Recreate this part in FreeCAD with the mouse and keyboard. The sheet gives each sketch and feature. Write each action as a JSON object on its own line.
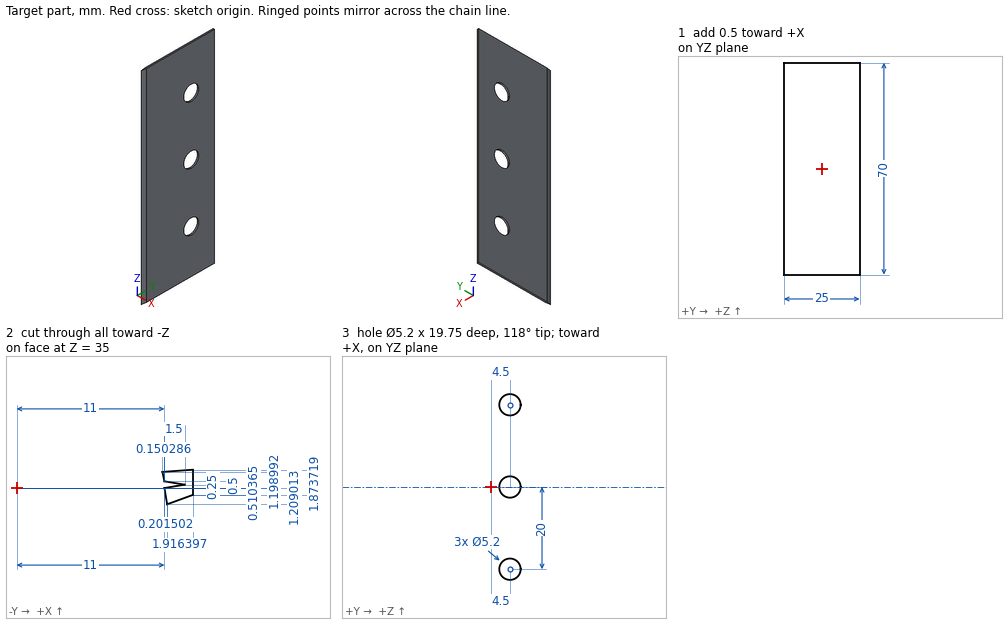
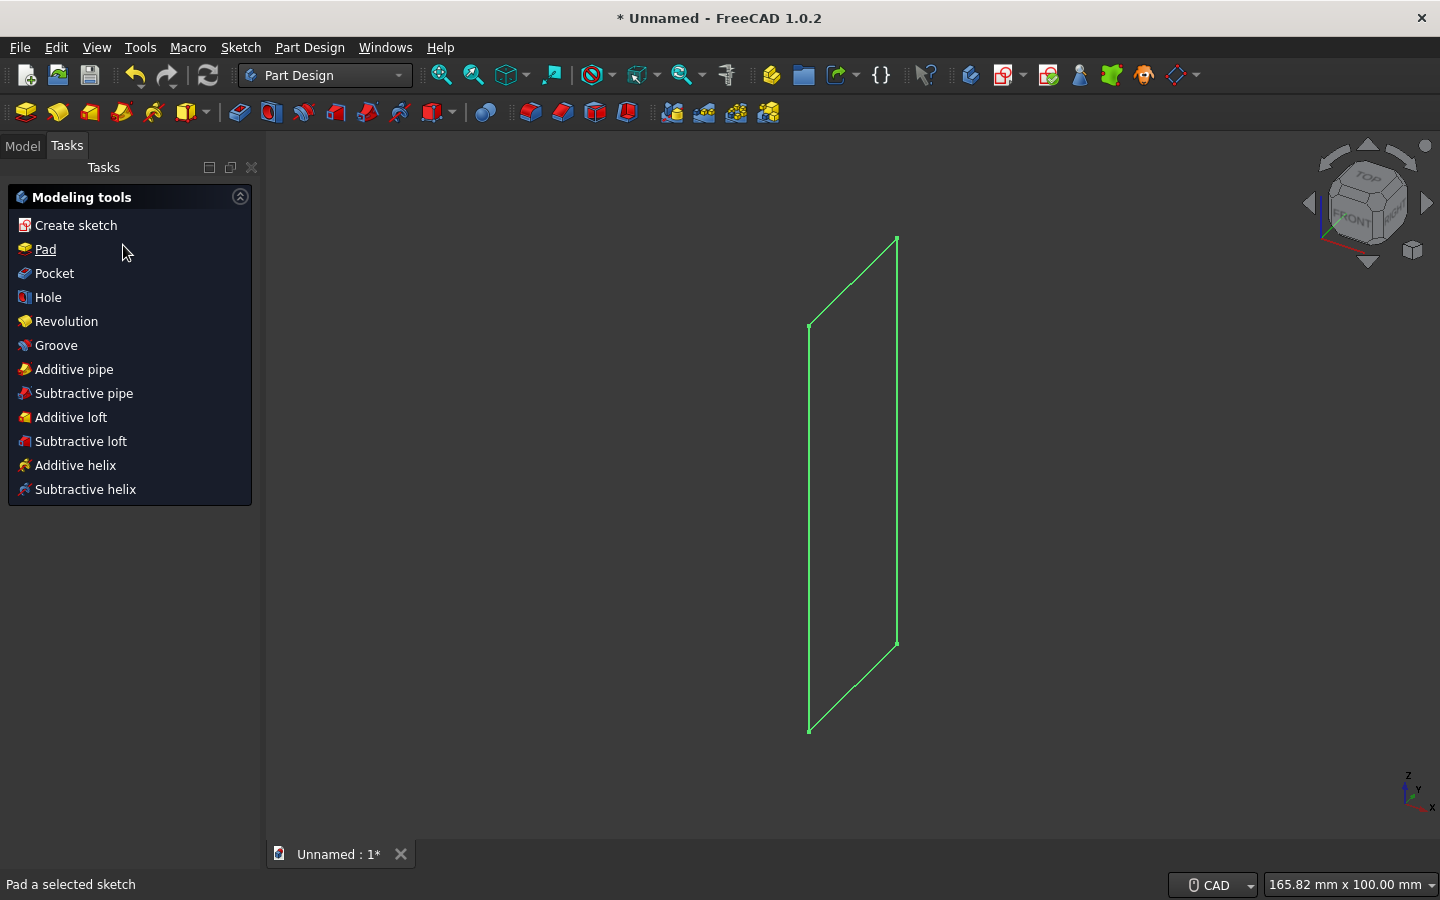
{"action": "left_click", "coordinate": [26, 112]}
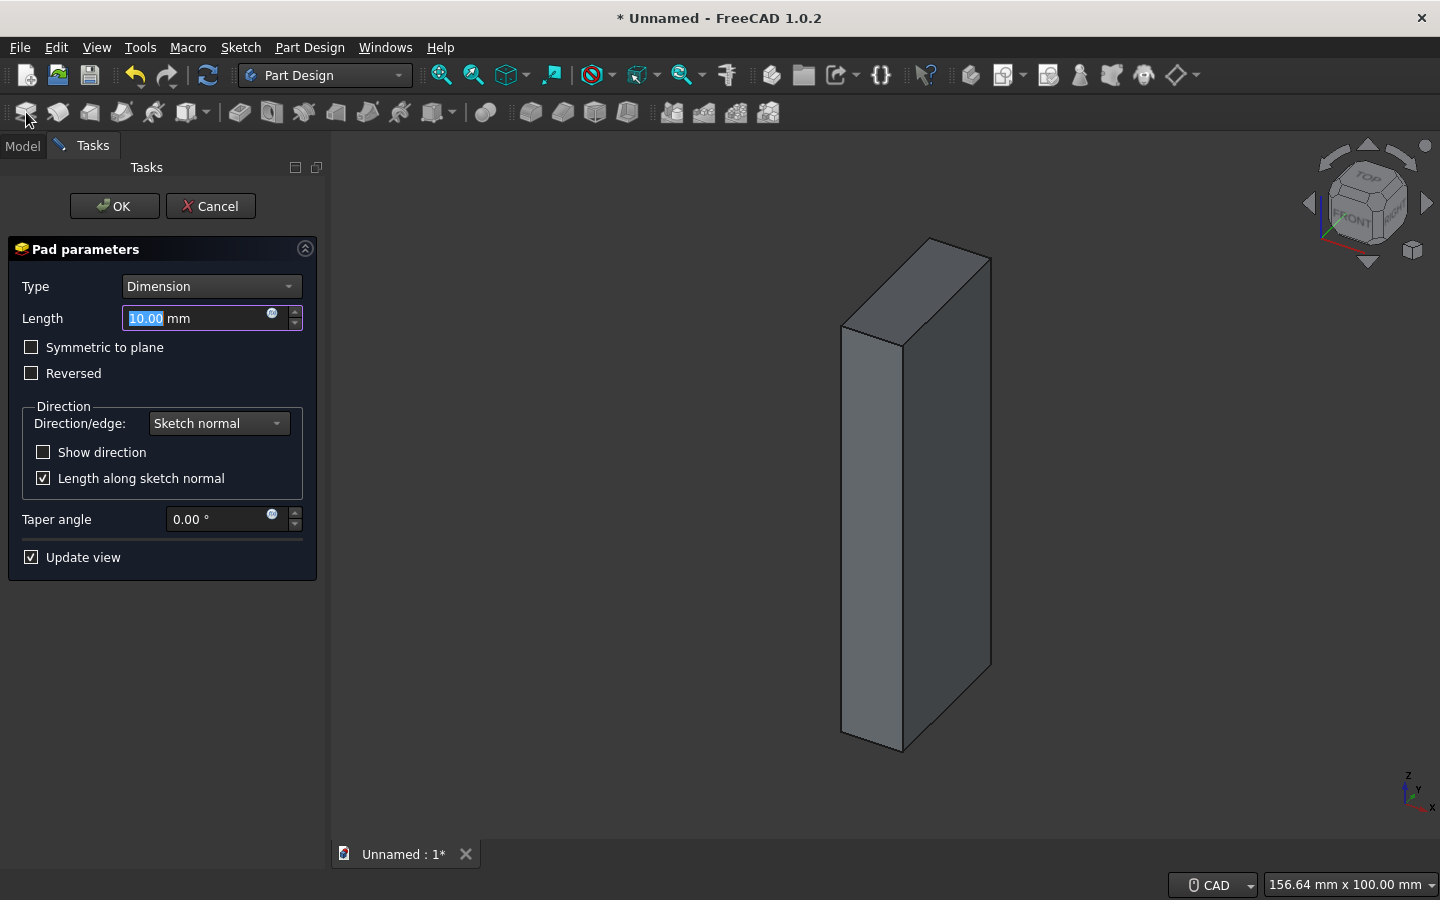
{"action": "type", "text": "0.5"}
{"action": "key", "text": "Tab"}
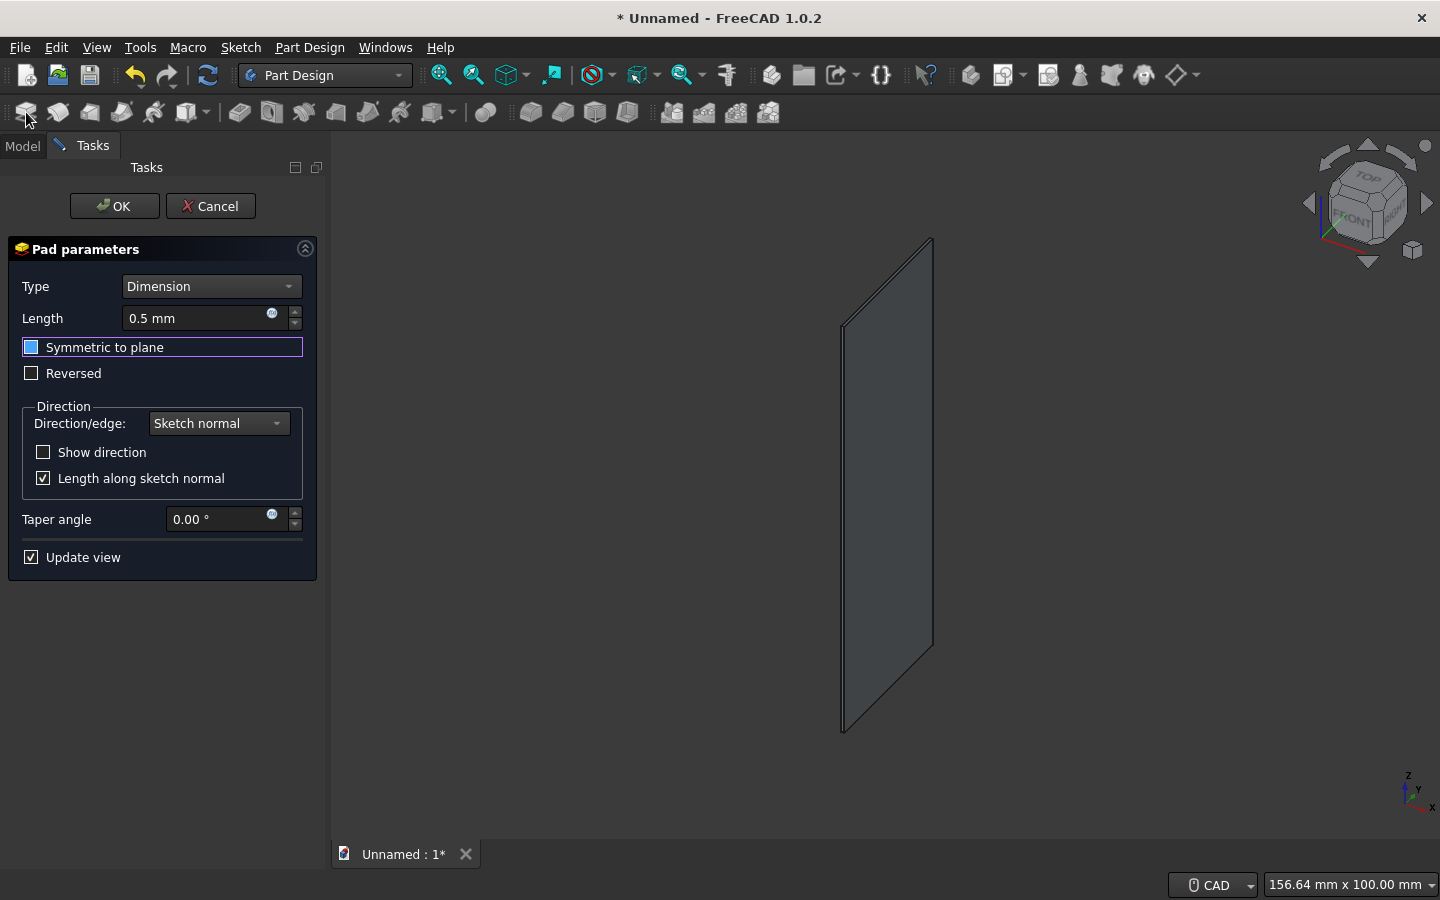
{"action": "left_click", "coordinate": [115, 206]}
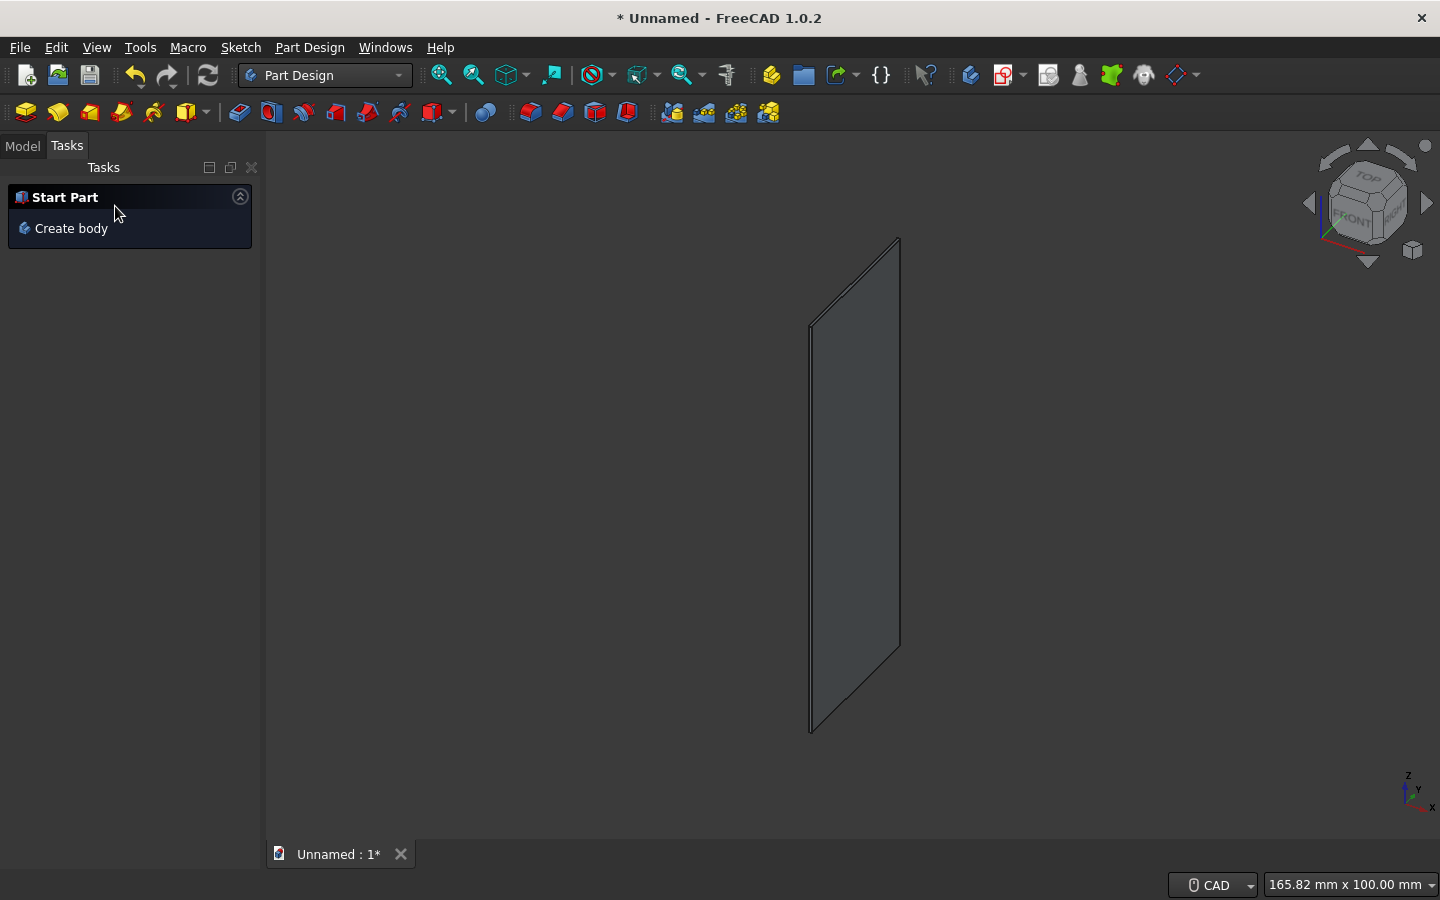
{"action": "scroll", "coordinate": [892, 244], "scroll_direction": "up", "scroll_amount": 10}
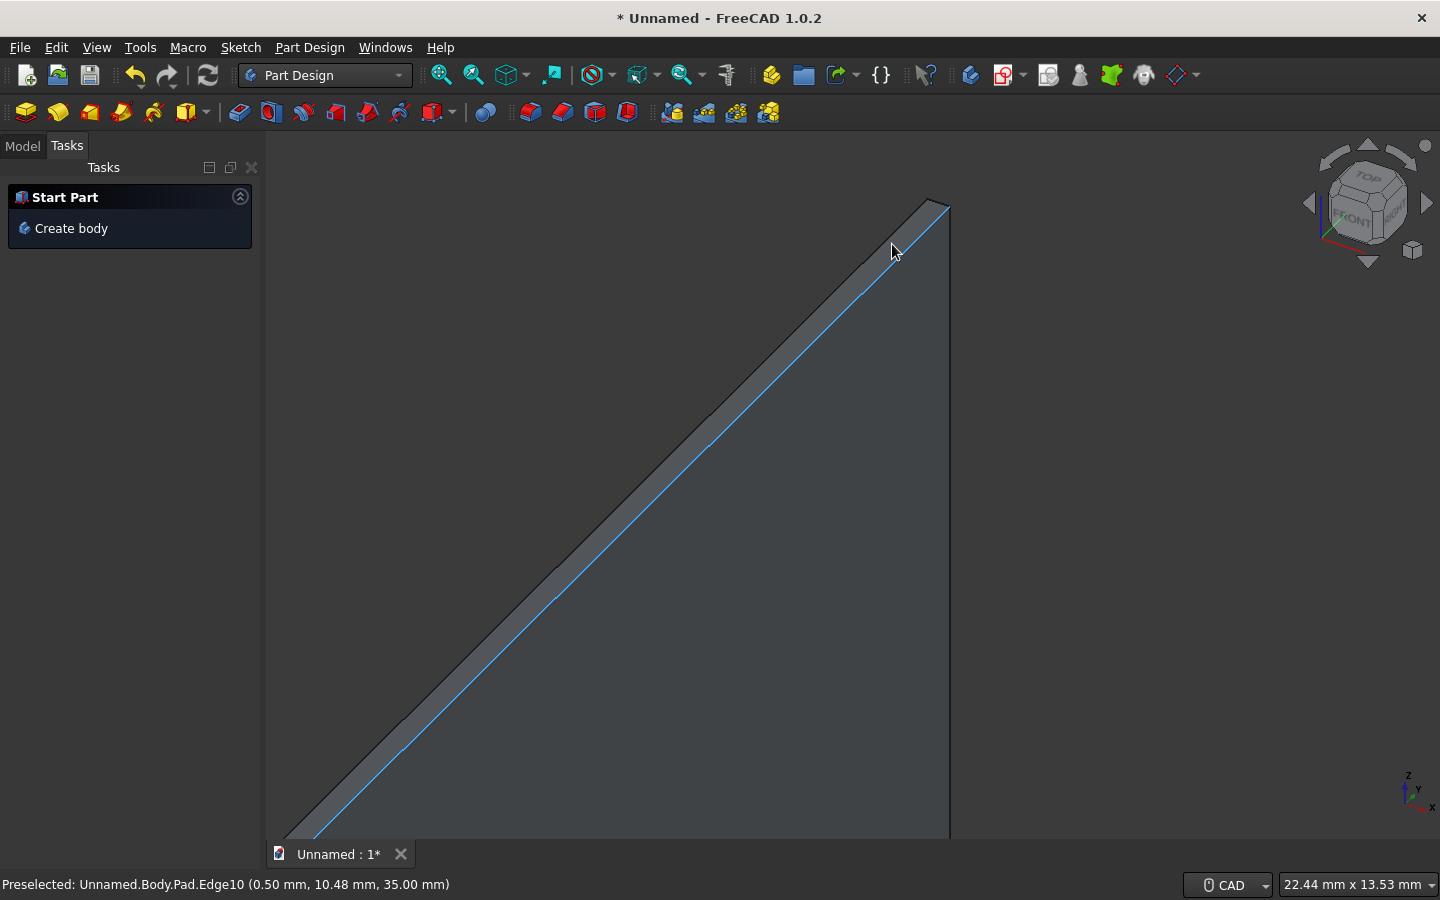
{"action": "left_click", "coordinate": [892, 248]}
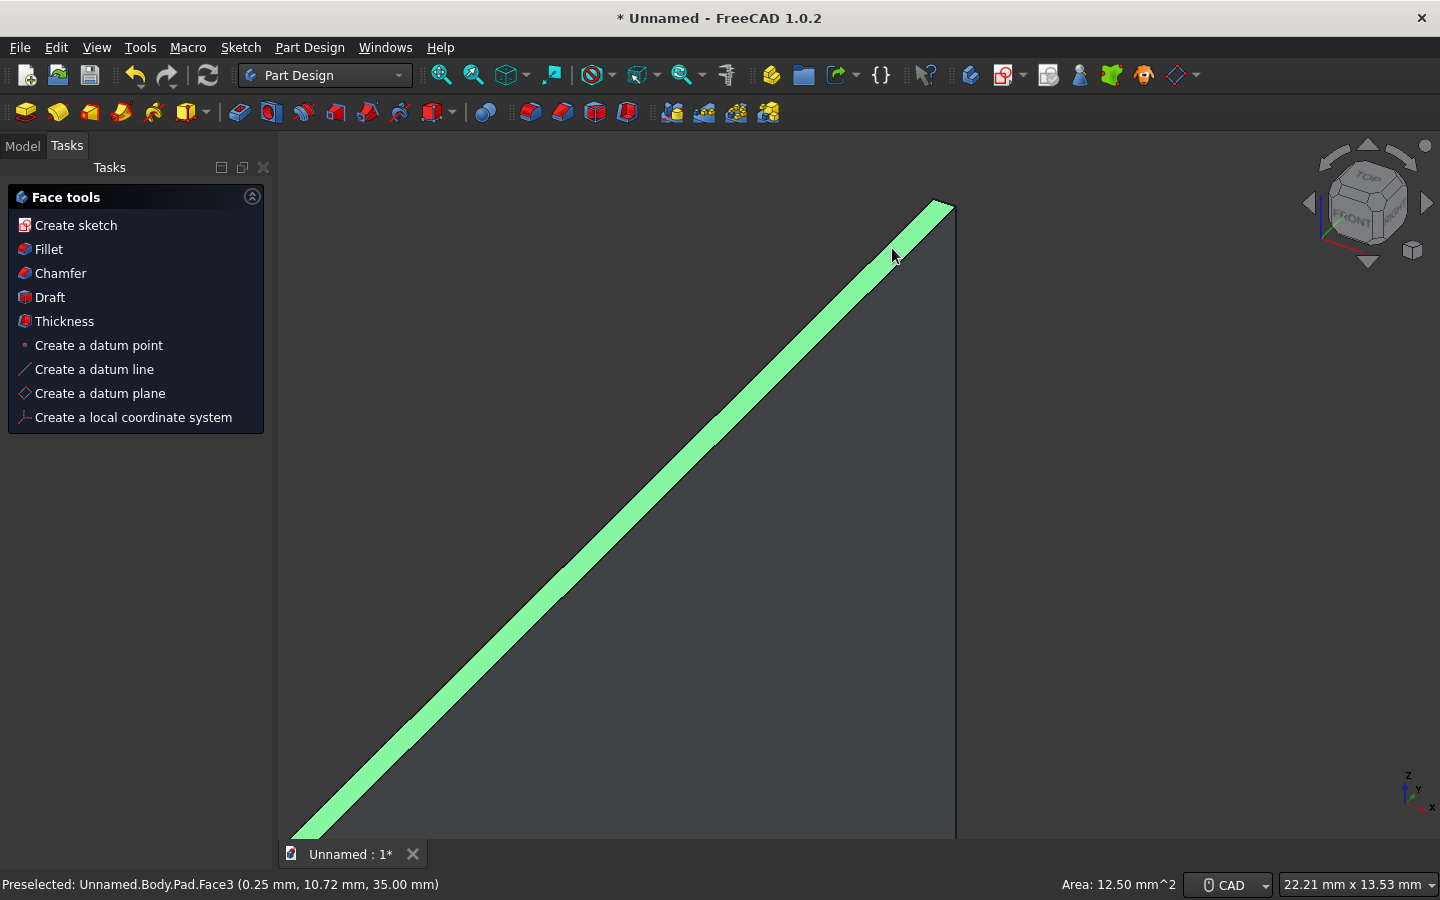
{"action": "left_click", "coordinate": [1004, 76]}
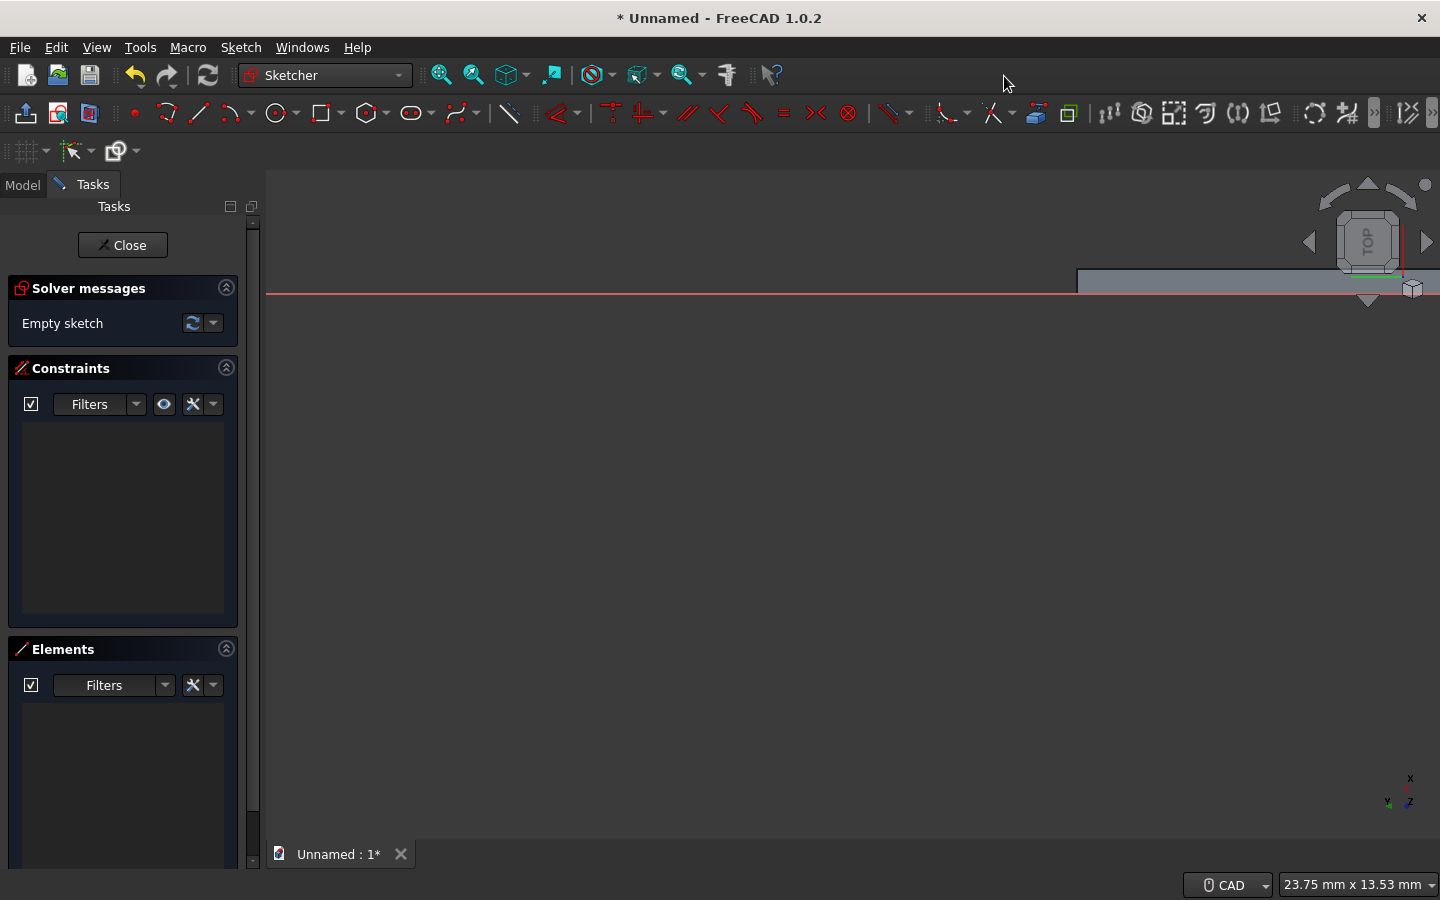
{"action": "scroll", "coordinate": [784, 504], "scroll_direction": "down", "scroll_amount": 5}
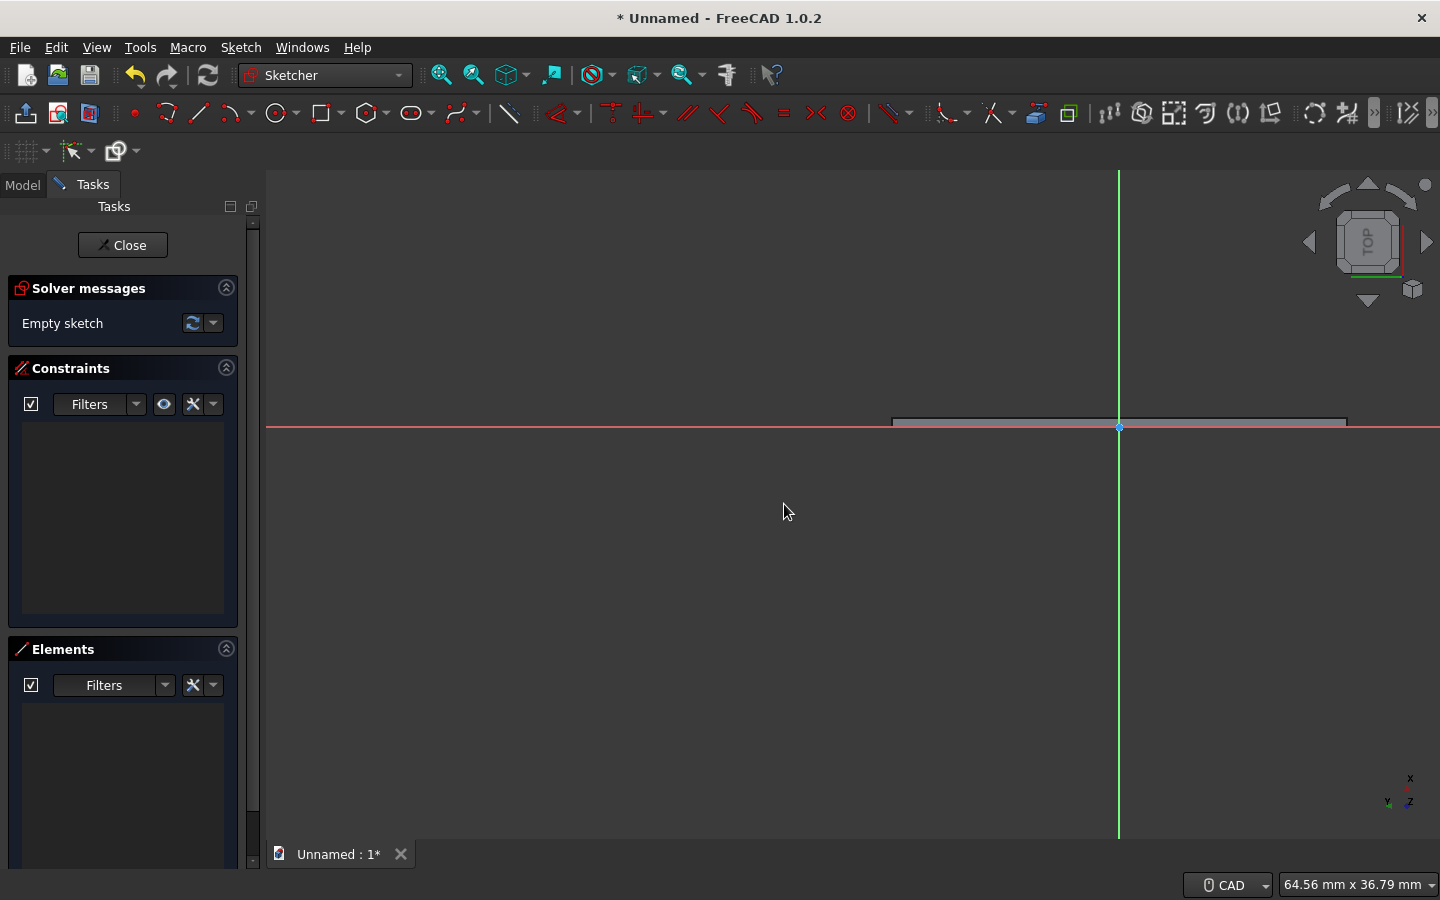
{"action": "scroll", "coordinate": [784, 504], "scroll_direction": "down", "scroll_amount": 5}